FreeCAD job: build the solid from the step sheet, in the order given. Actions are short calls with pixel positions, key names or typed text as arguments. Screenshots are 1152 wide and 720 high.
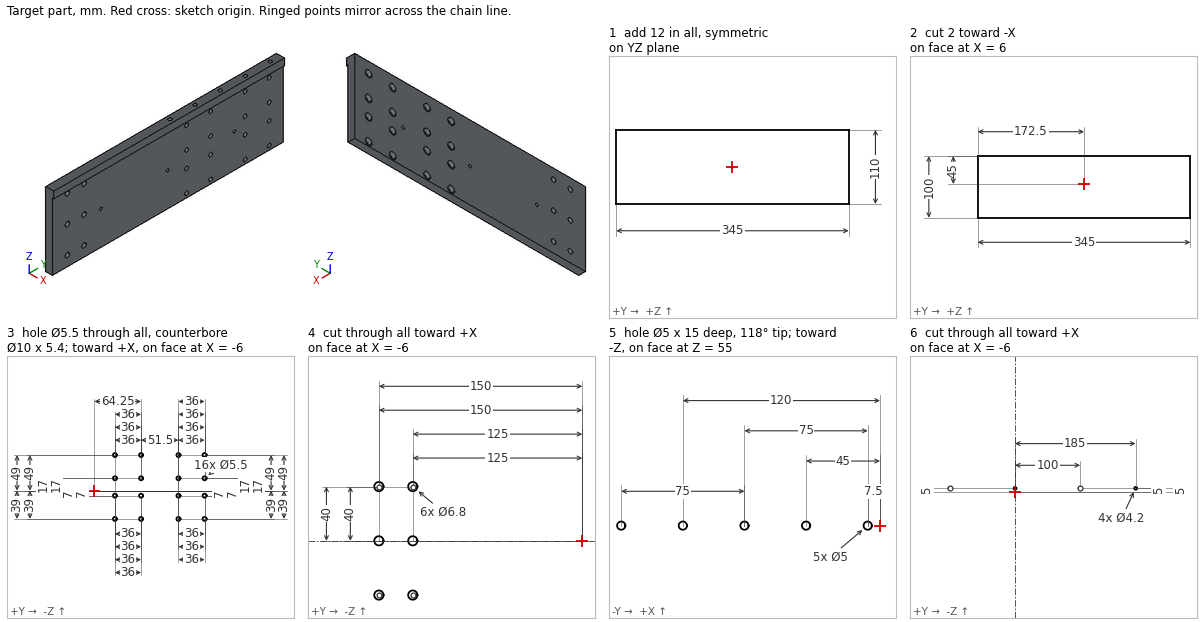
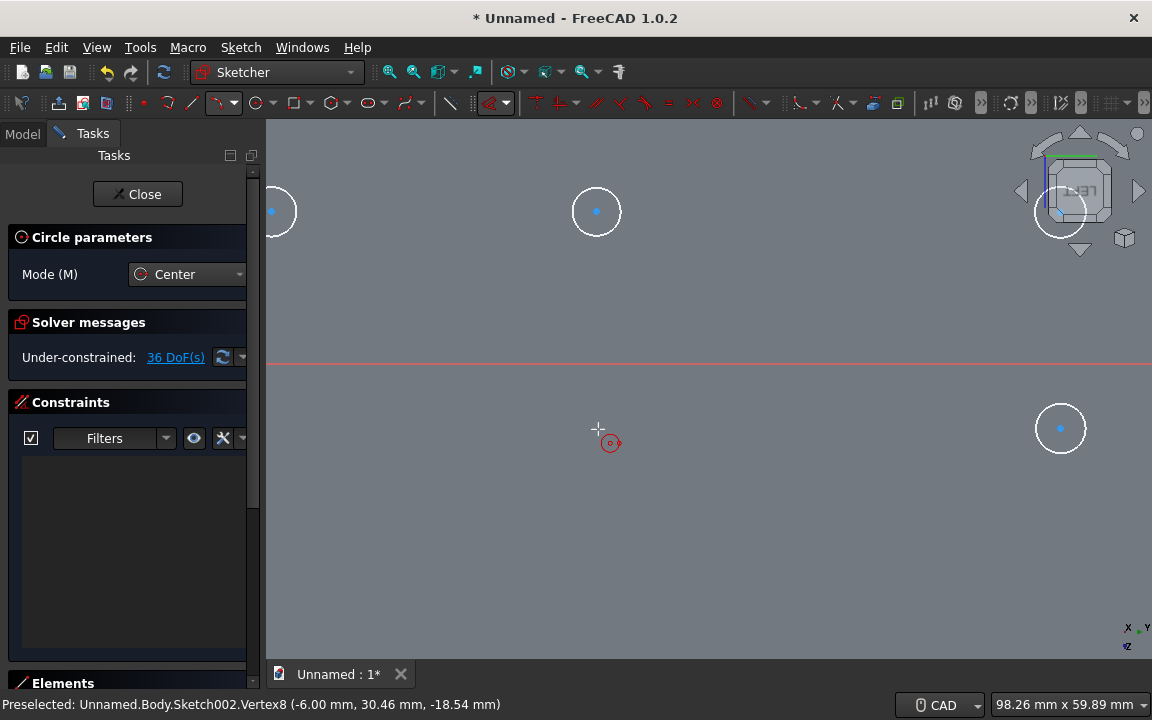
click(596, 427)
click(614, 410)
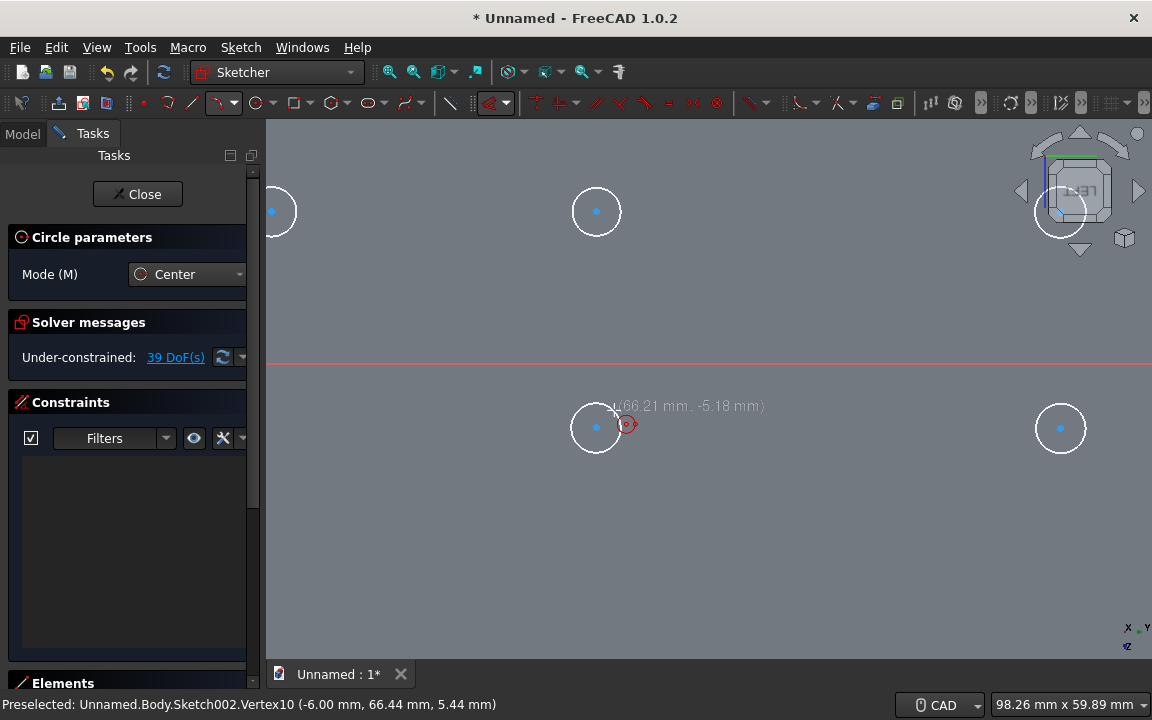
scroll(598, 430, down, 5)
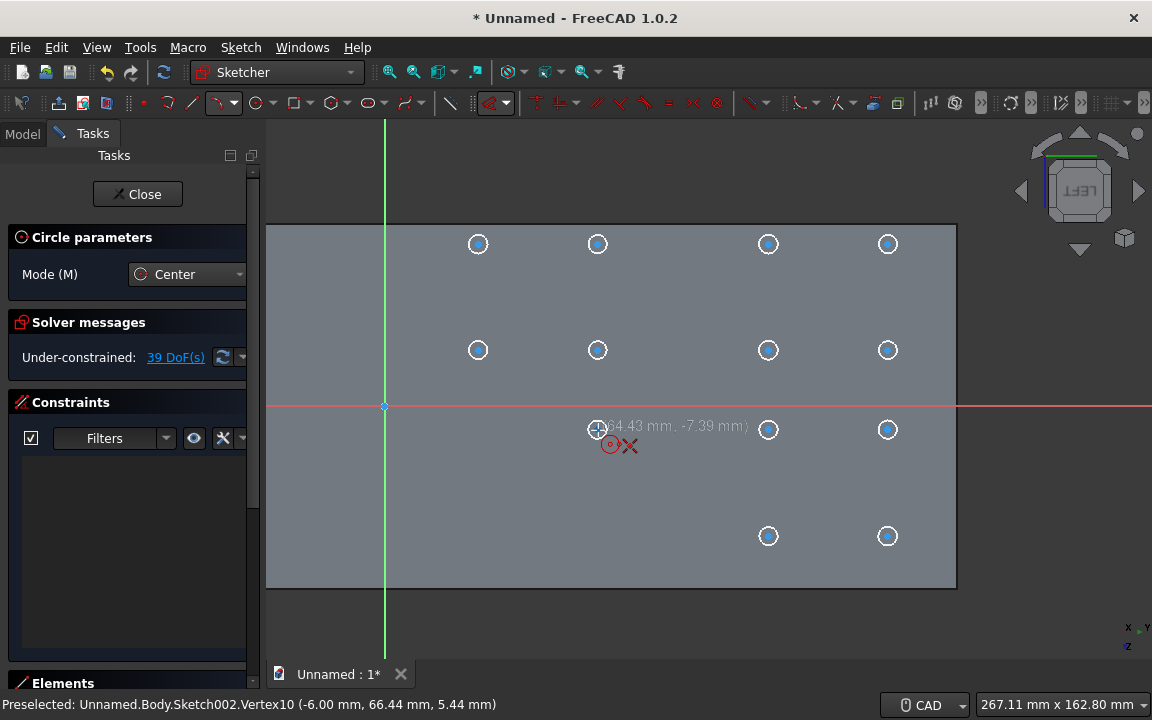
scroll(478, 429, up, 5)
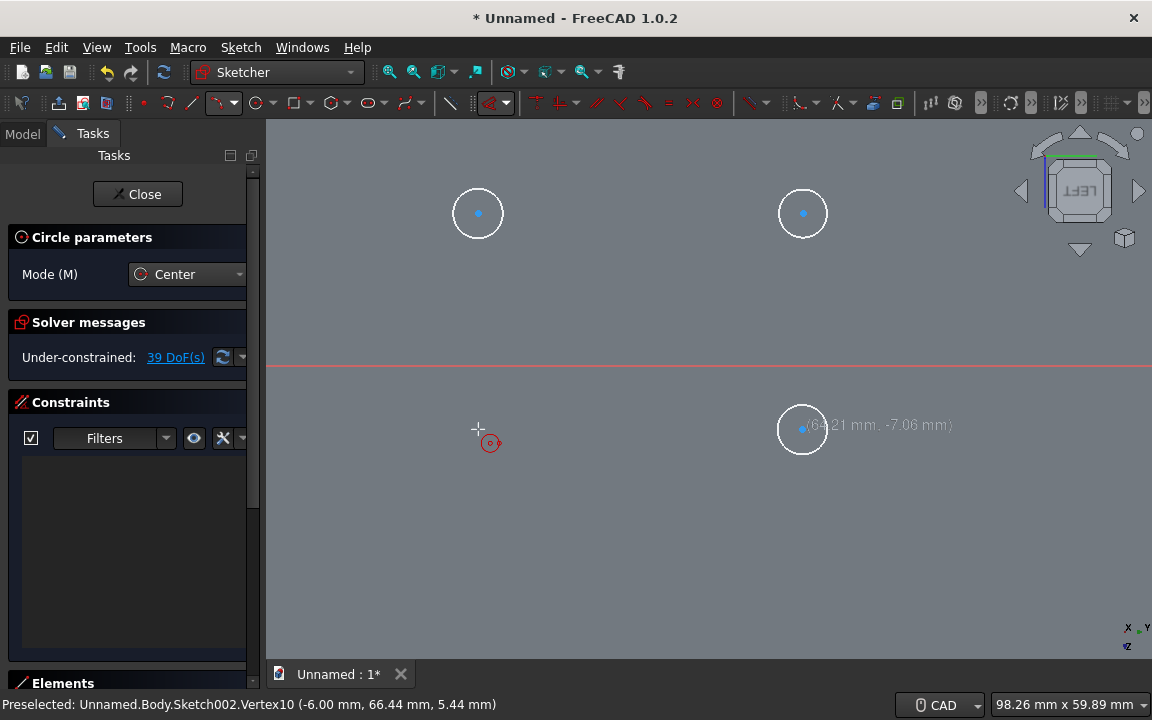
click(478, 429)
click(496, 412)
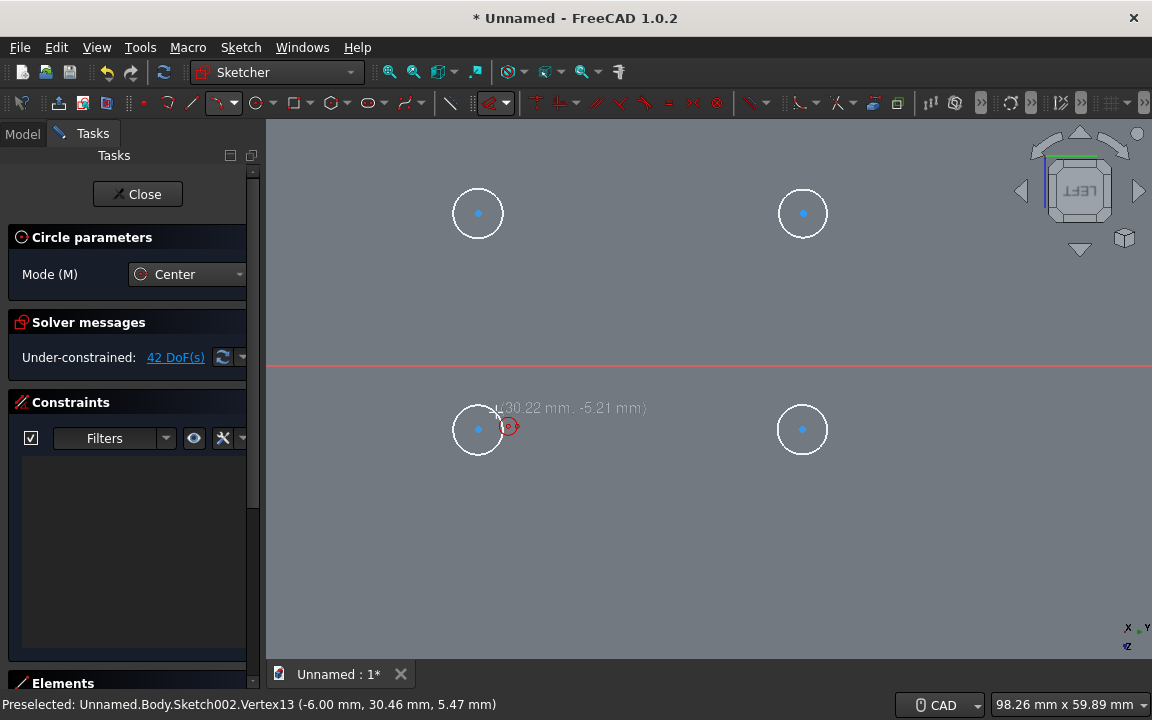
scroll(478, 429, down, 5)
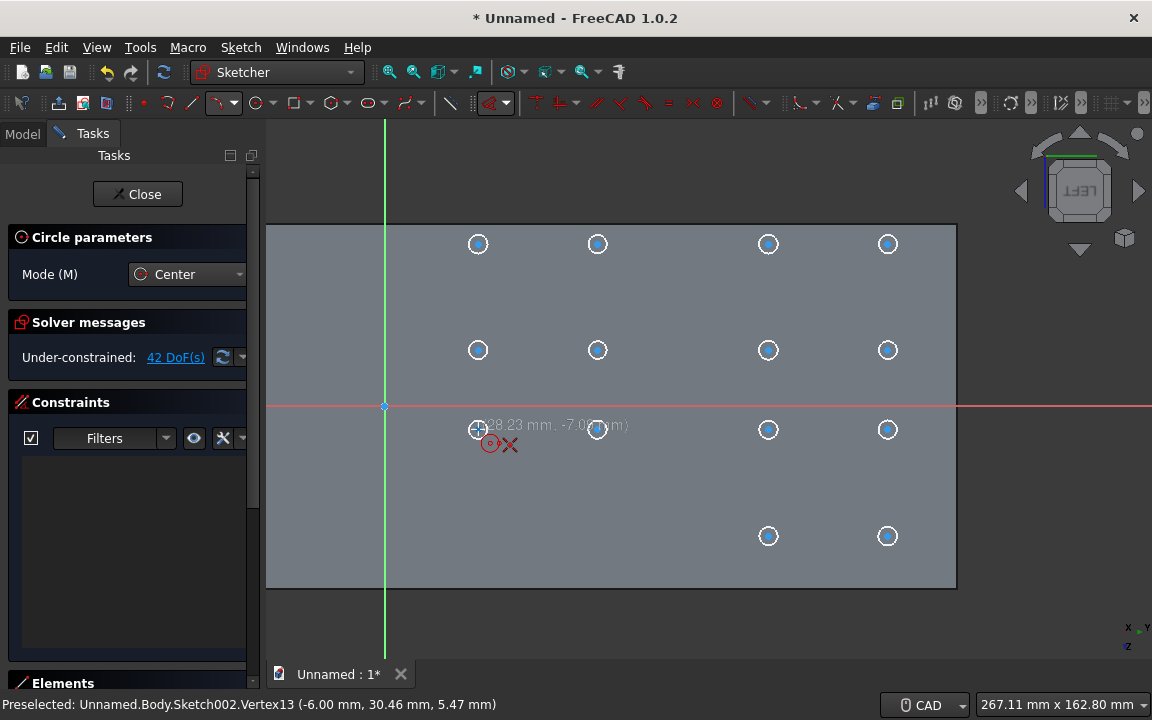
scroll(598, 536, up, 5)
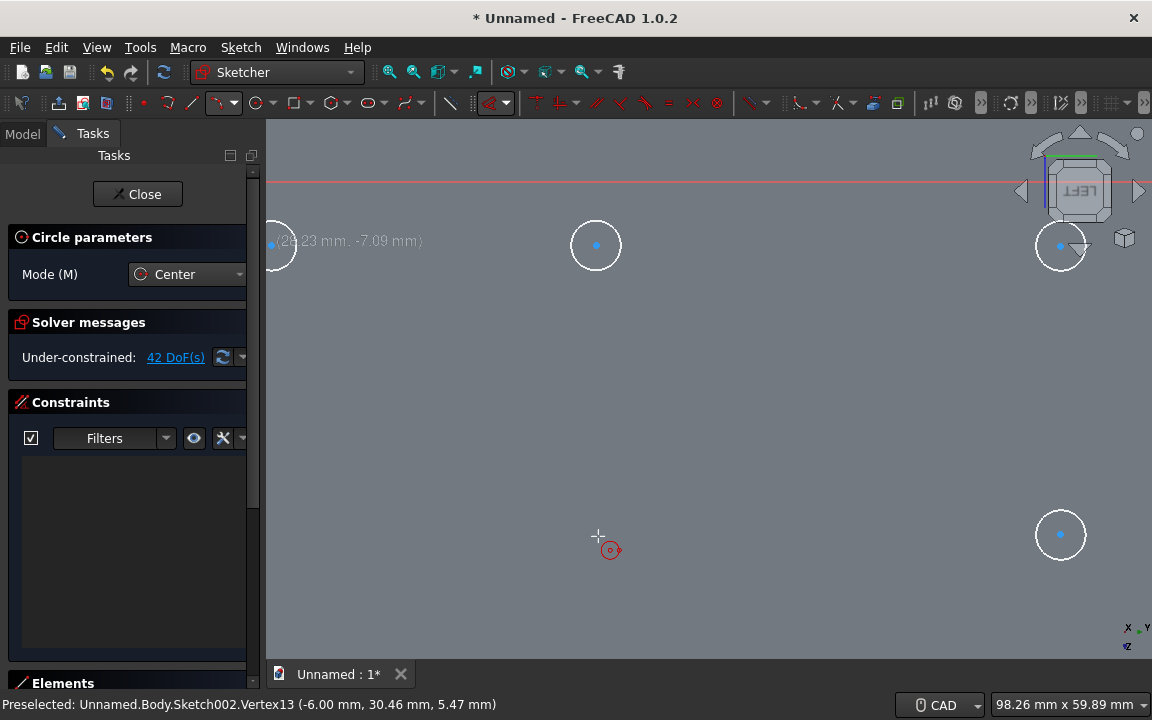
click(596, 534)
click(614, 516)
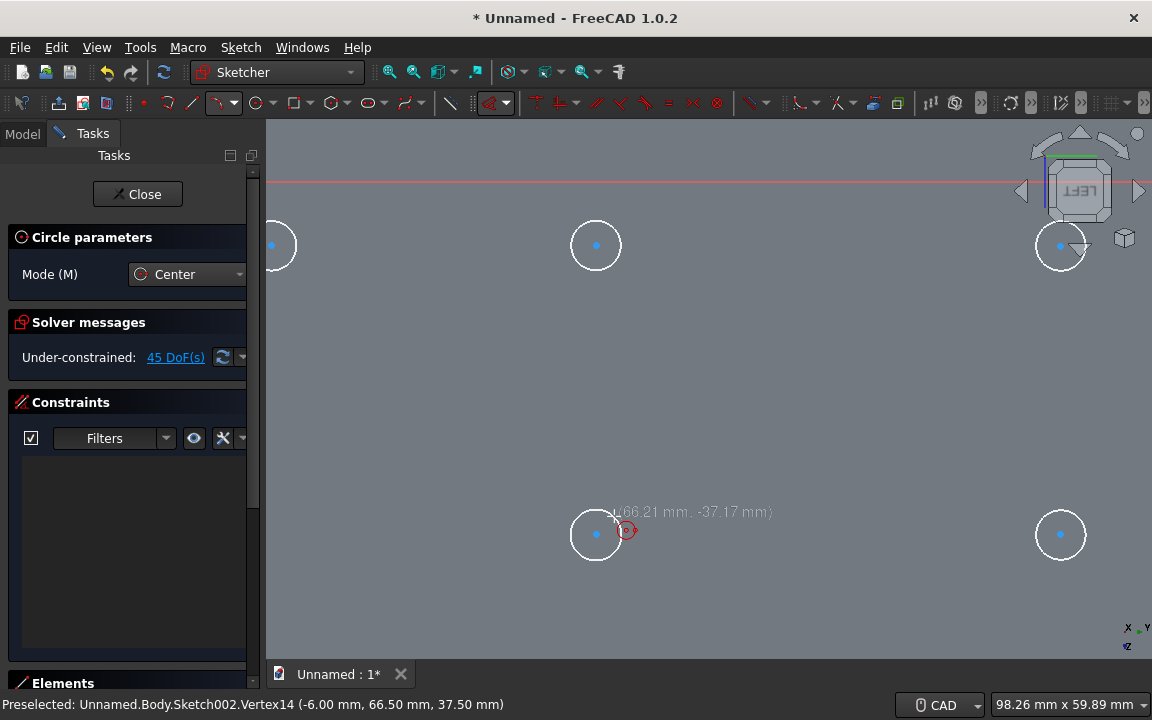
scroll(598, 536, down, 5)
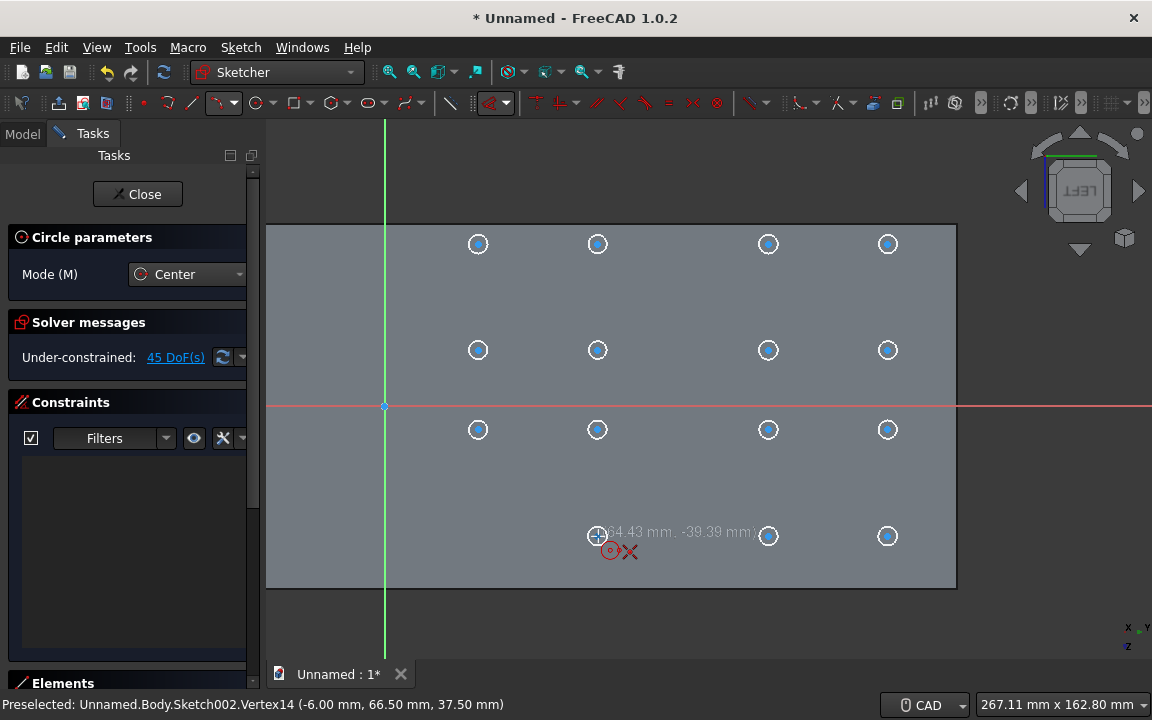
scroll(478, 536, up, 5)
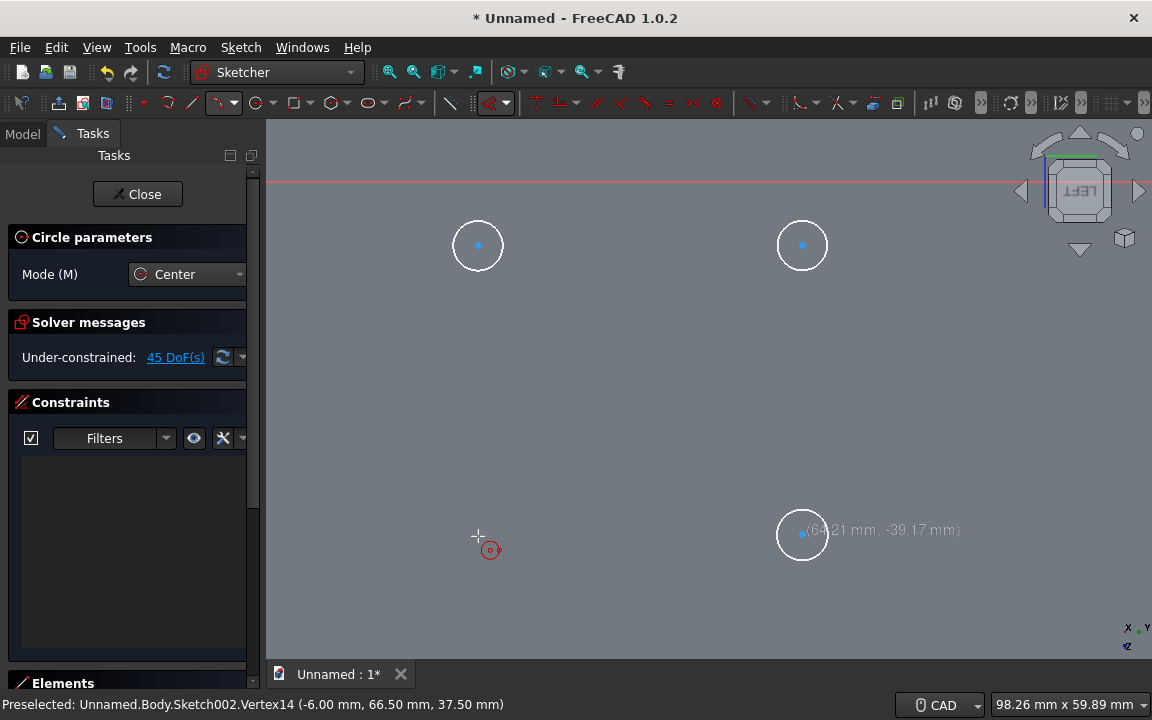
click(478, 534)
click(496, 516)
key(Escape)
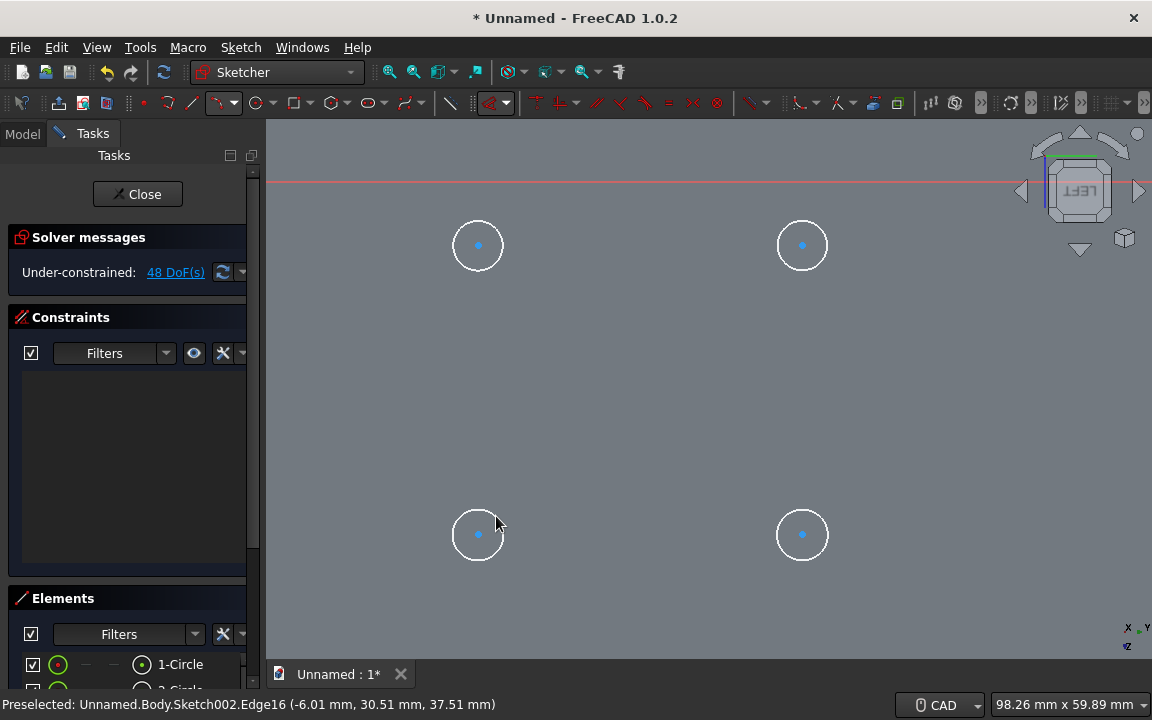
scroll(478, 536, down, 5)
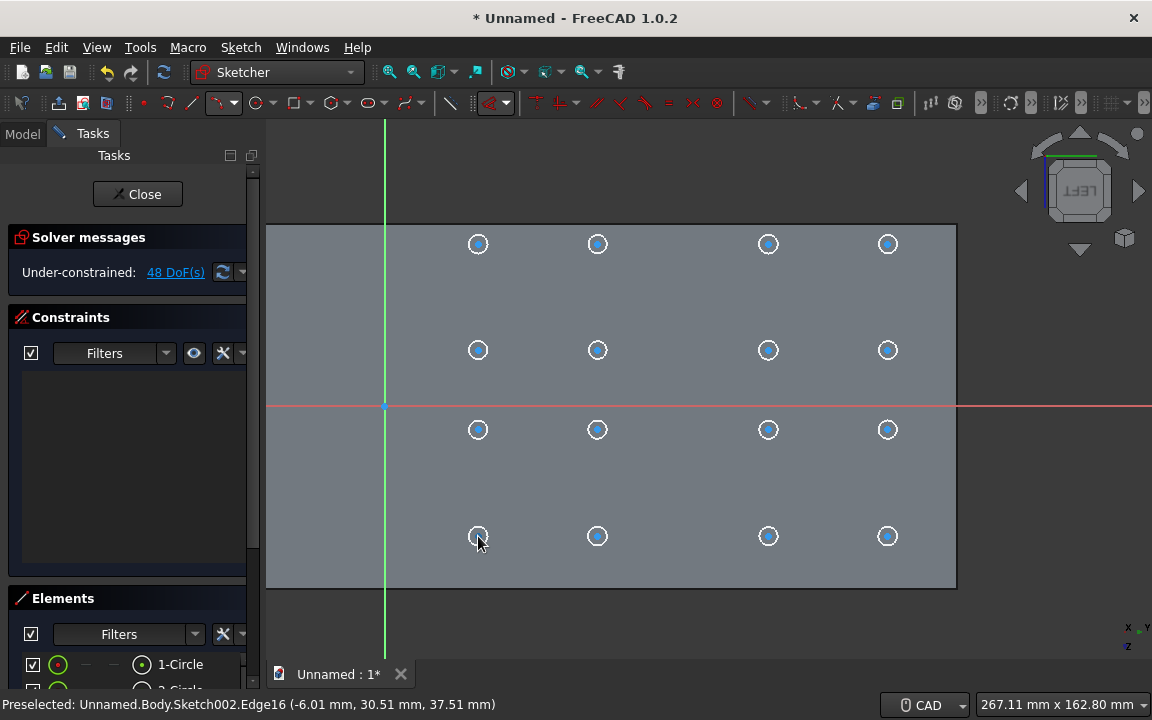
scroll(894, 238, up, 3)